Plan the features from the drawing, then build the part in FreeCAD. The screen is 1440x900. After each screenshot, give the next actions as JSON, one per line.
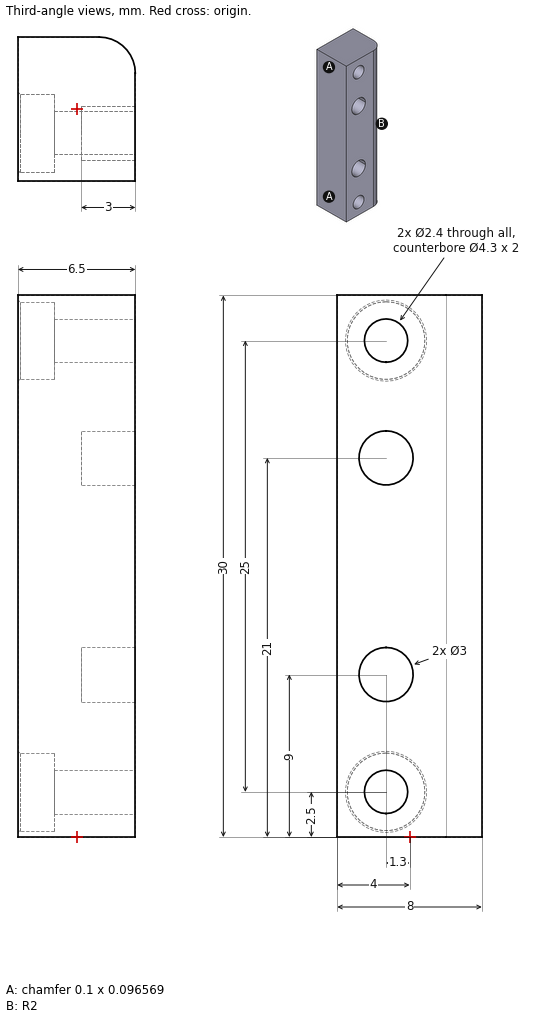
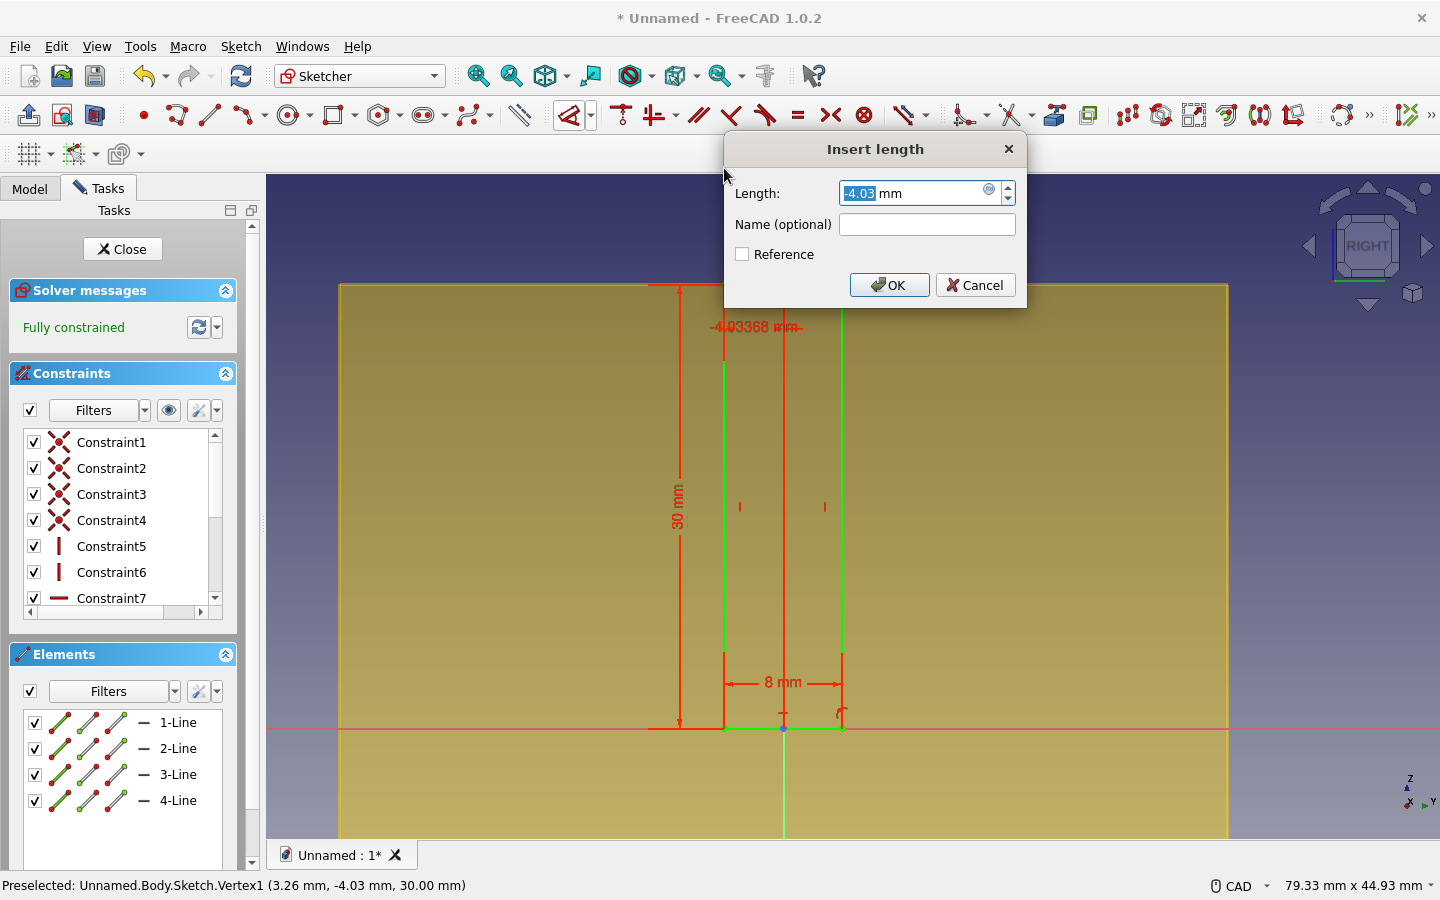
{"action": "type", "text": "-4"}
{"action": "key", "text": "Return"}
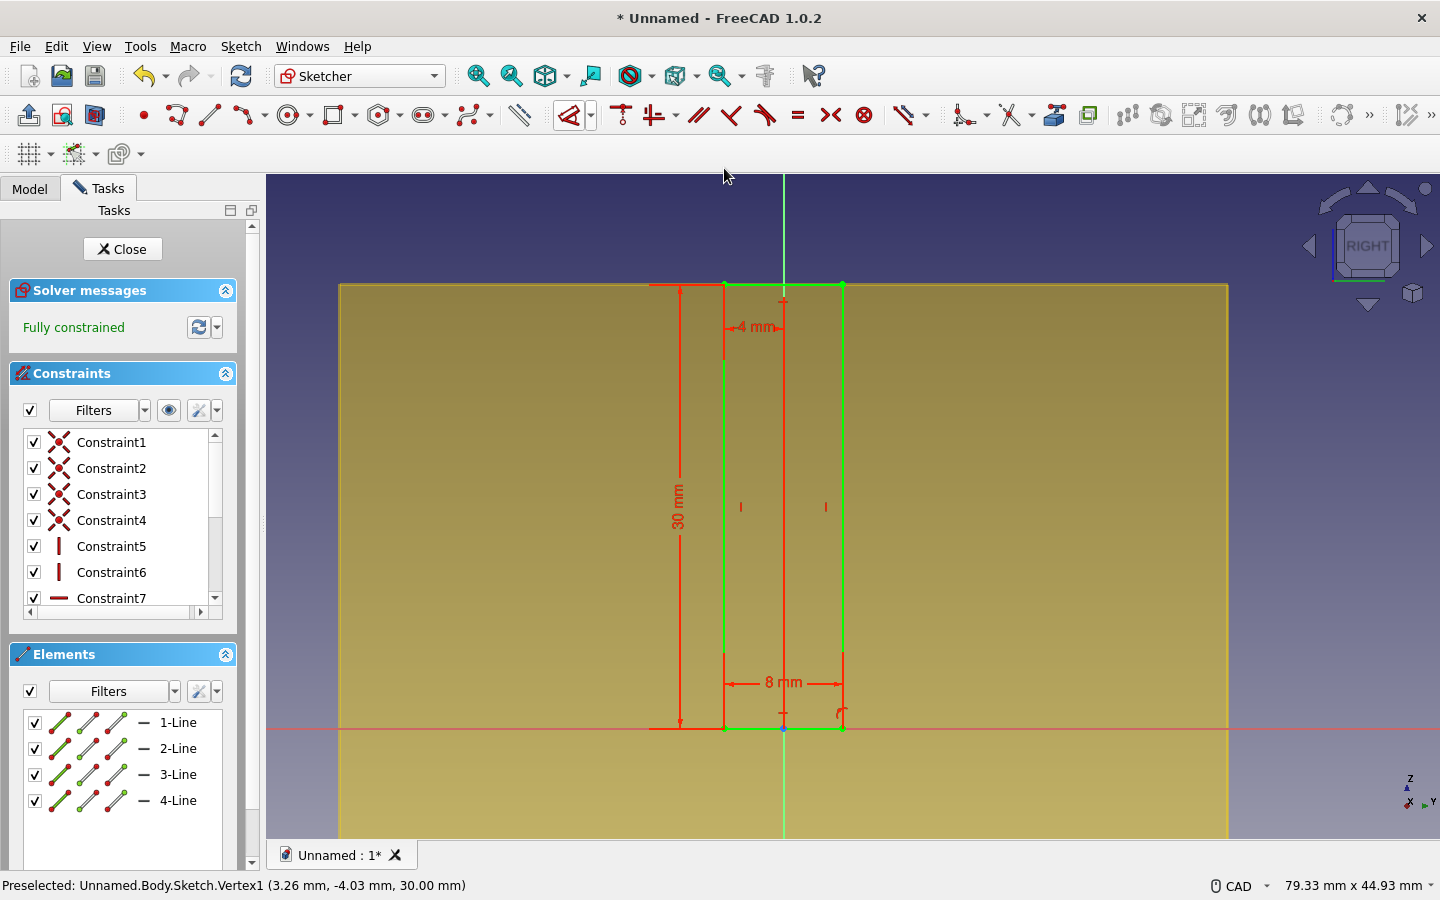
{"action": "left_click", "coordinate": [123, 249]}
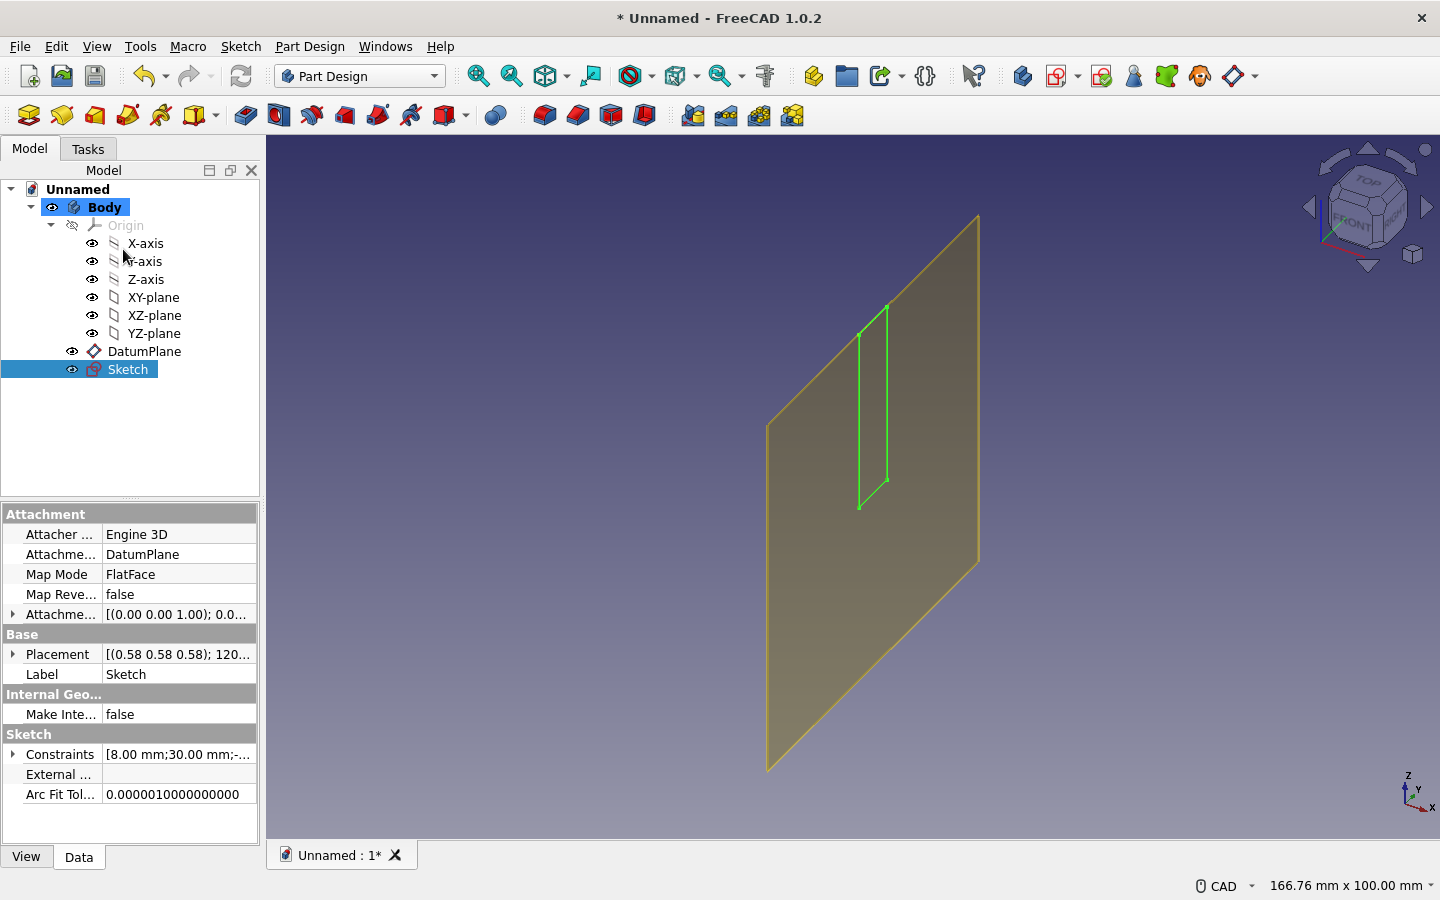
{"action": "left_click", "coordinate": [29, 116]}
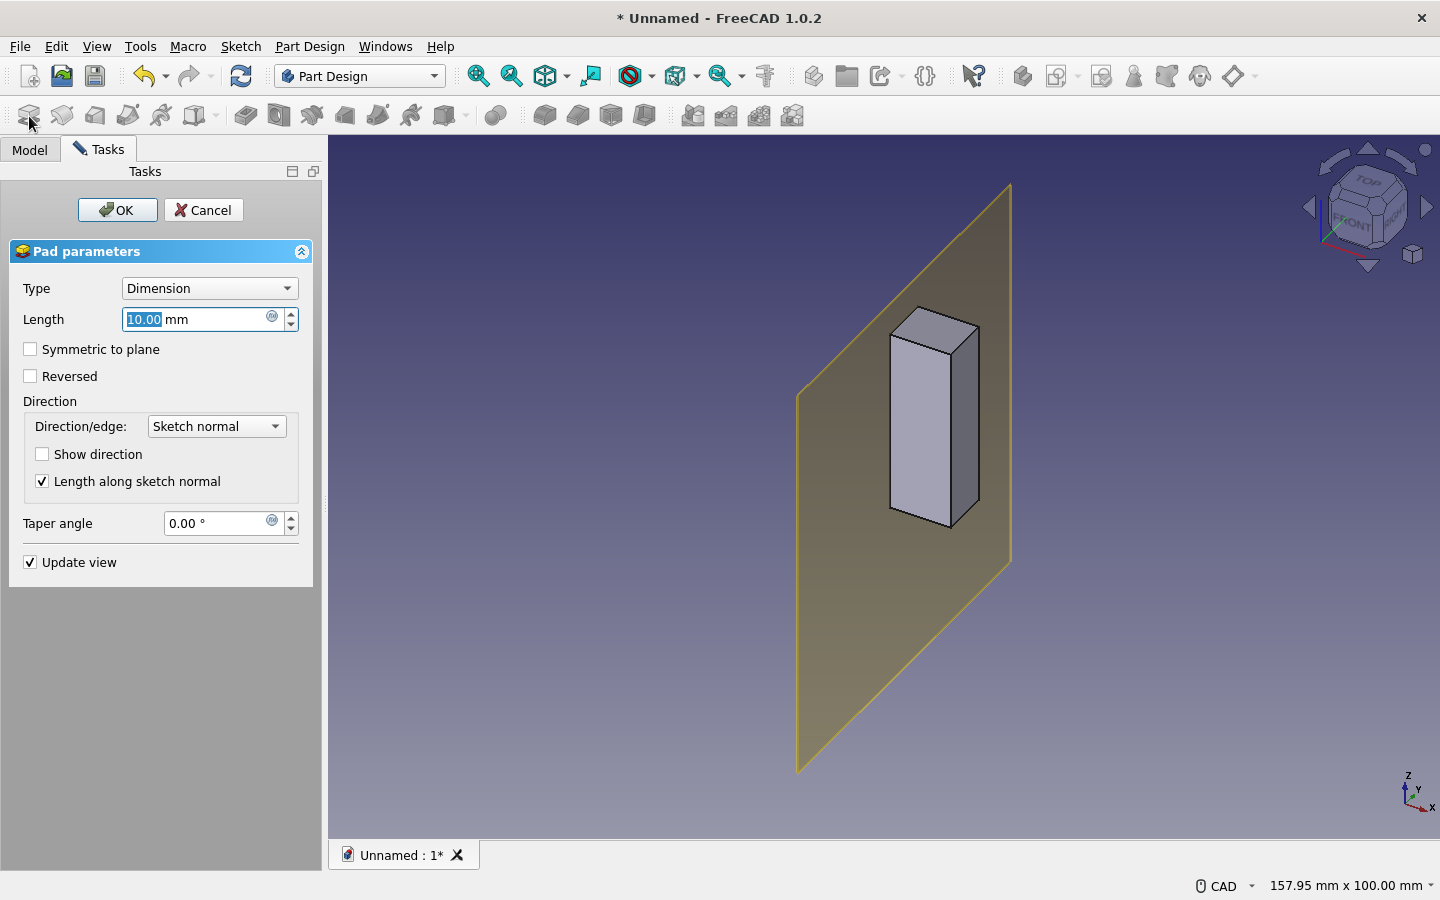
{"action": "type", "text": "6.5"}
{"action": "key", "text": "Tab"}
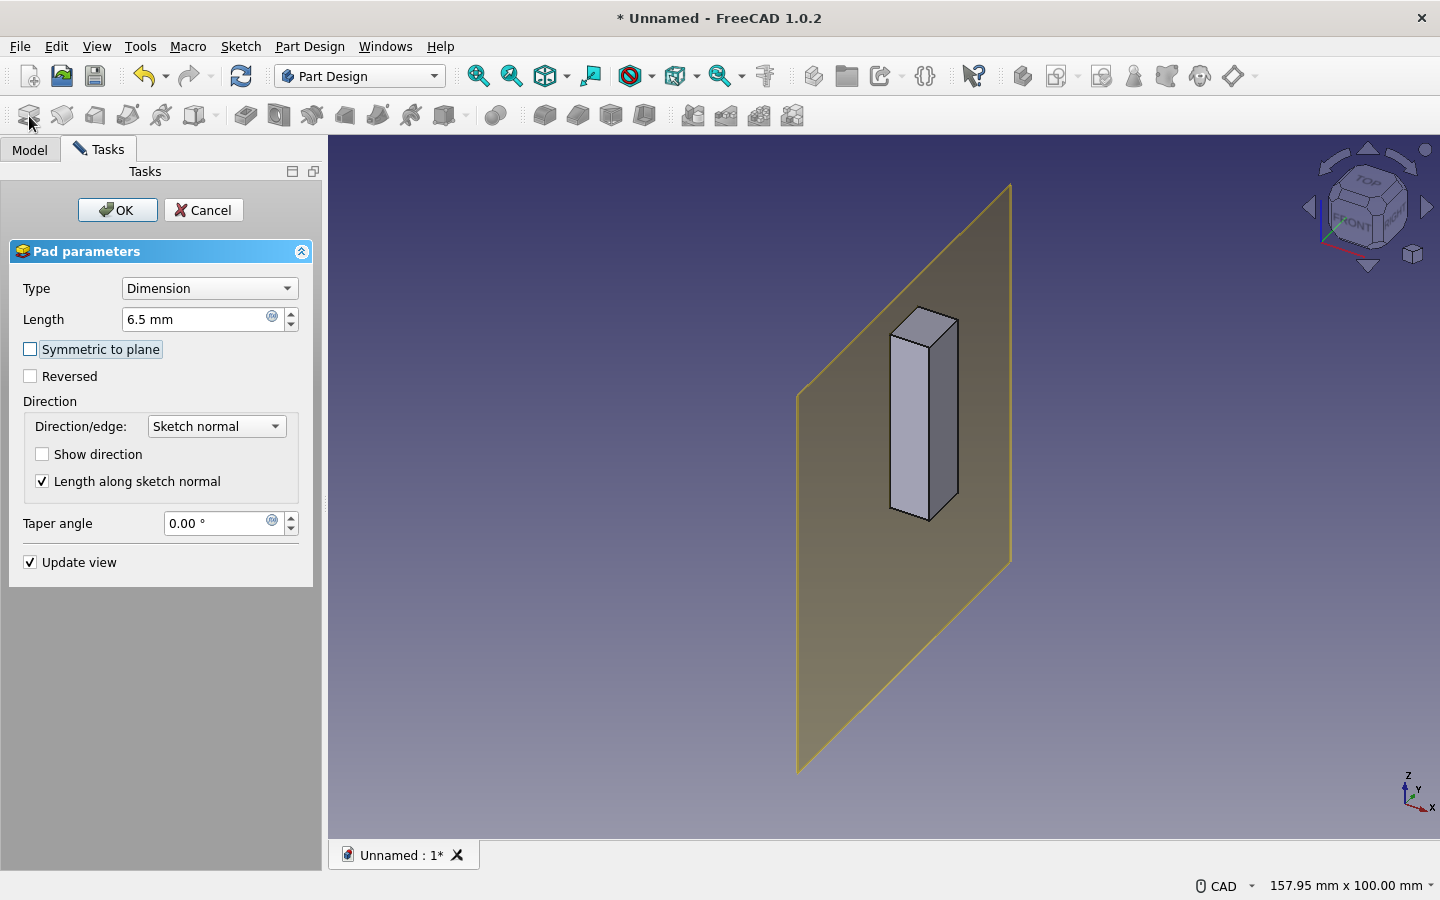
{"action": "left_click", "coordinate": [31, 376]}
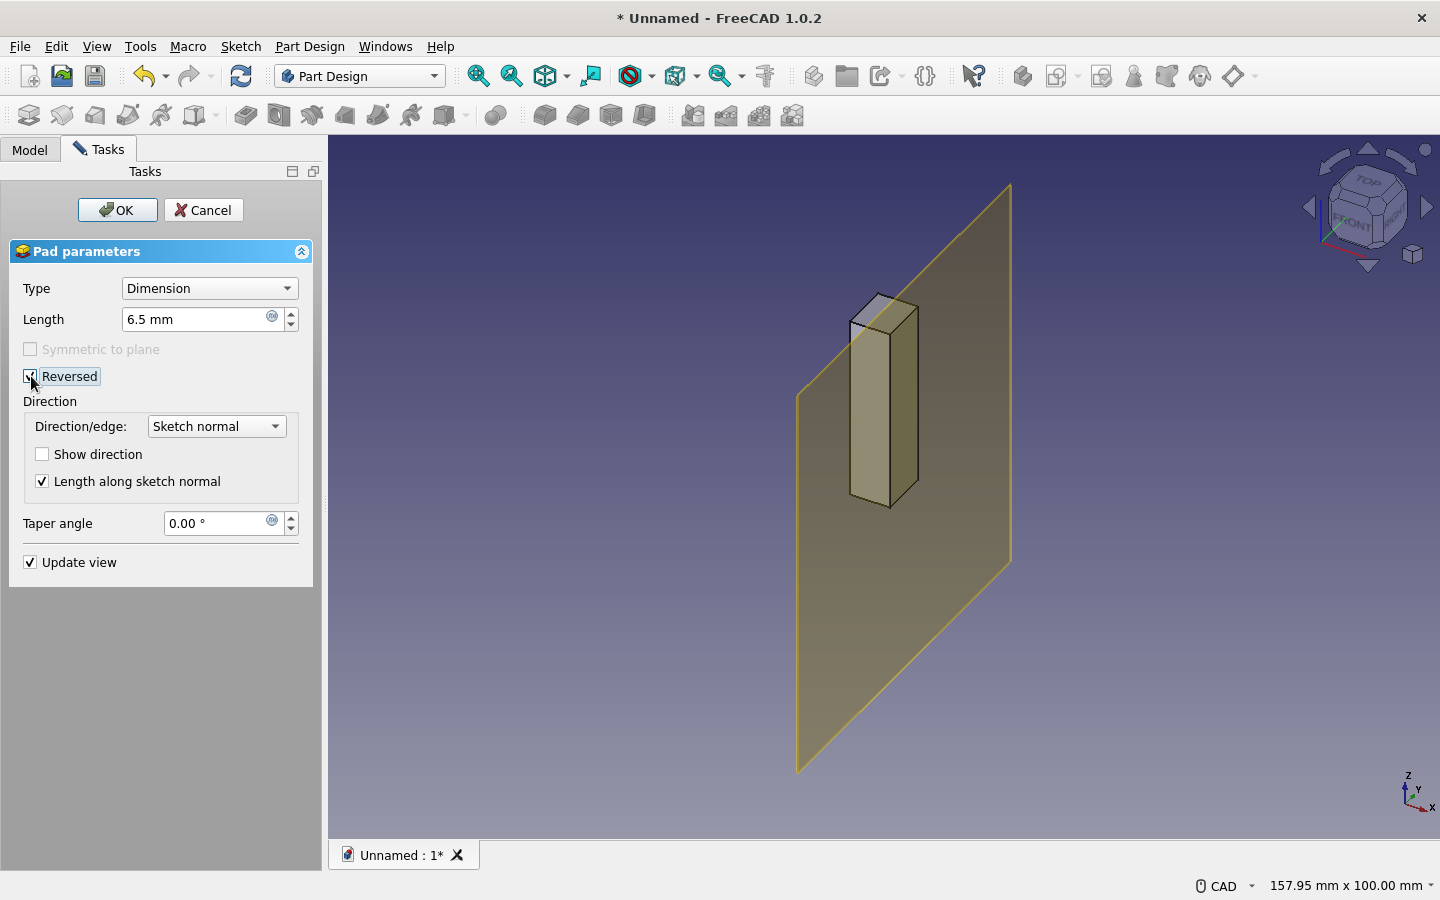
{"action": "left_click", "coordinate": [118, 210]}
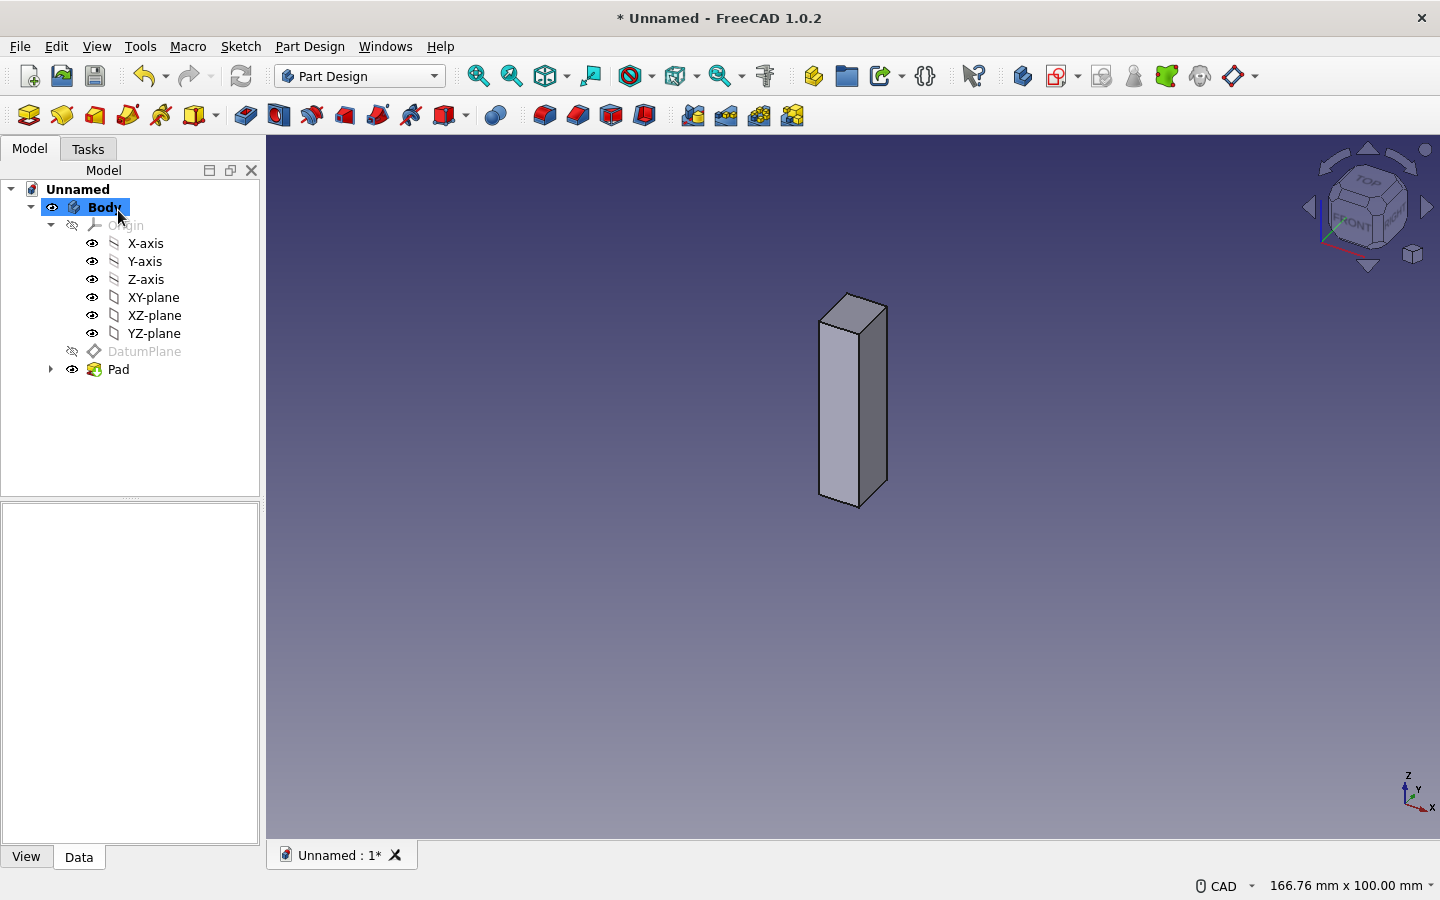
{"action": "left_click", "coordinate": [479, 76]}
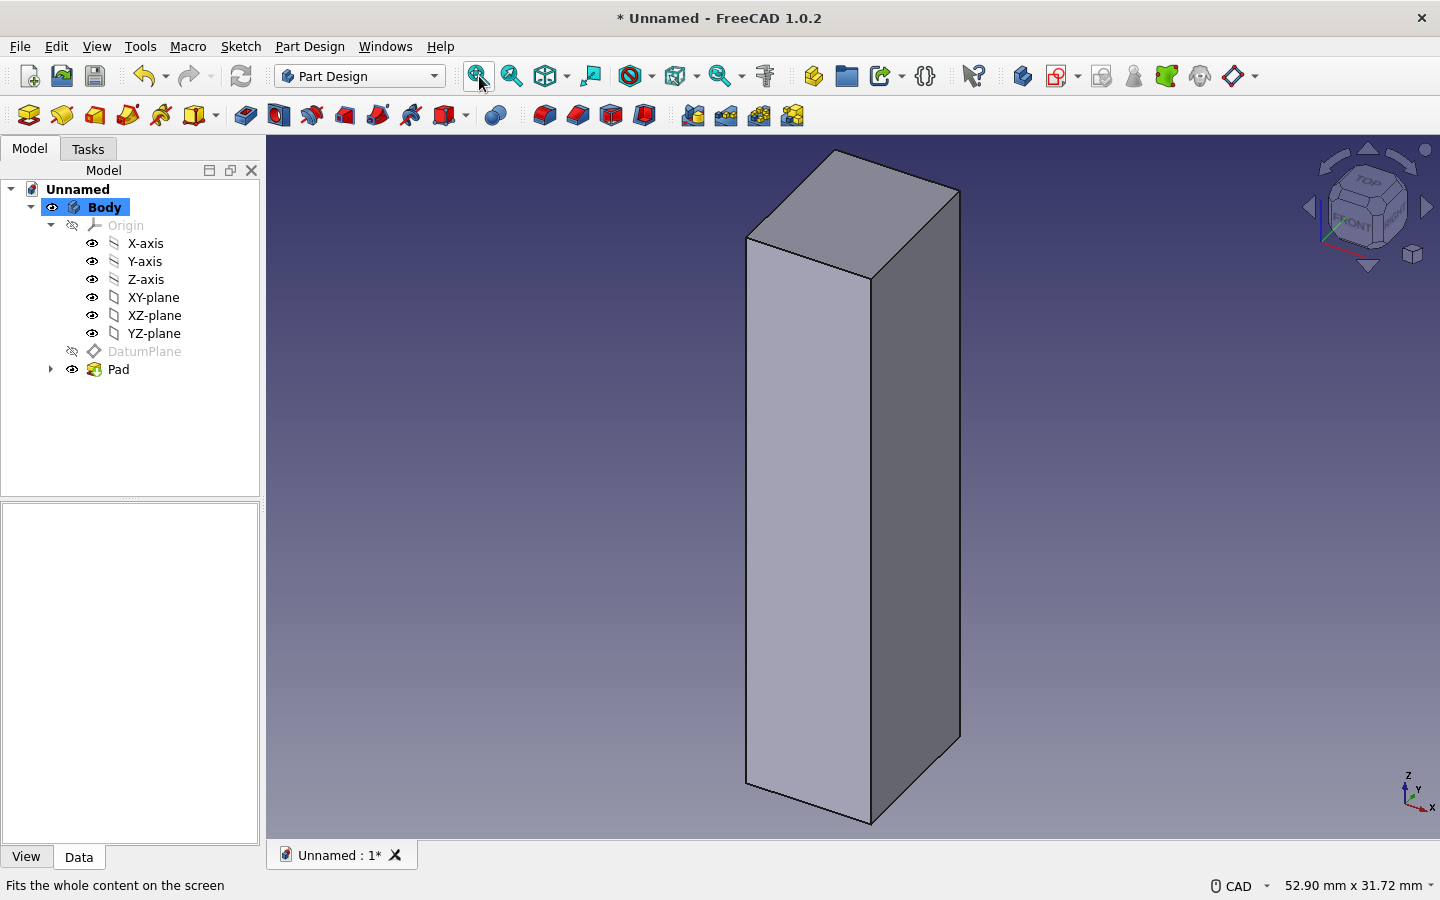
{"action": "left_click", "coordinate": [915, 429]}